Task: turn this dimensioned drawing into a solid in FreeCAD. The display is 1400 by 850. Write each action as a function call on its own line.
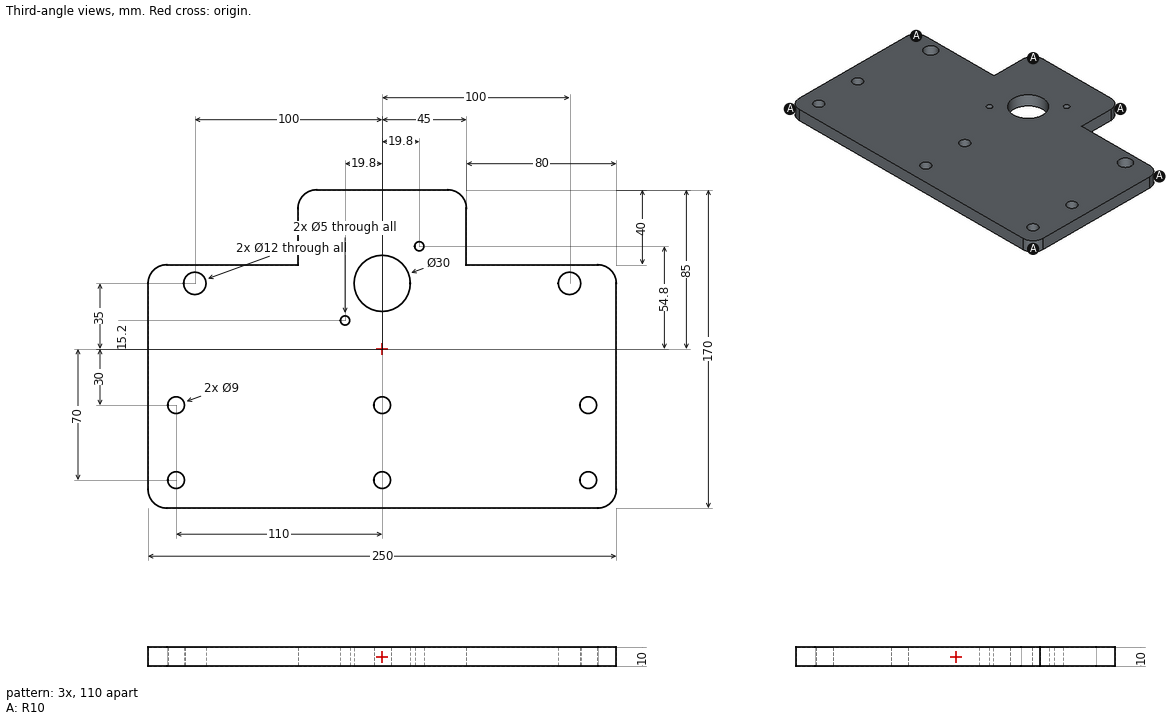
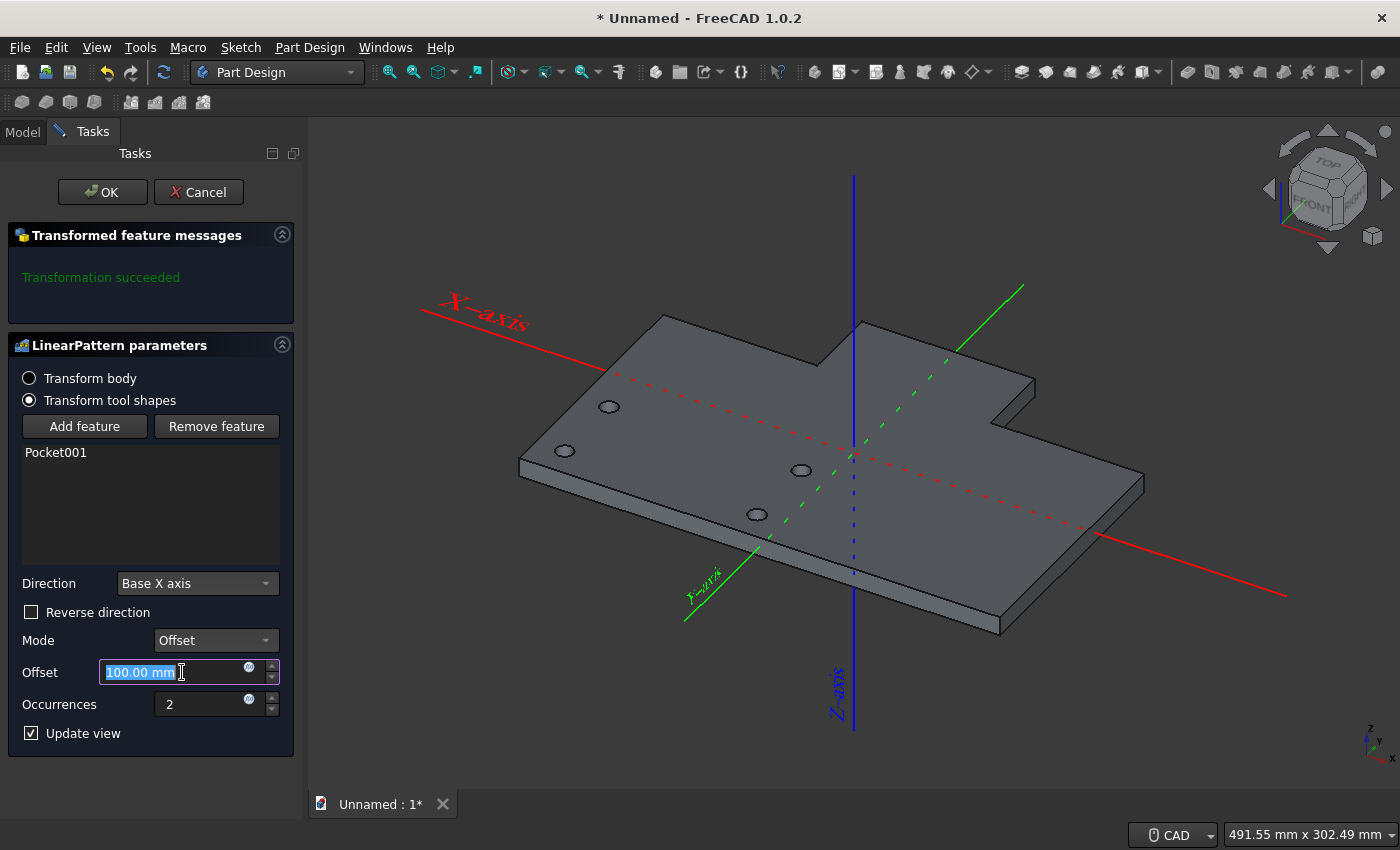
text(110)
key(Tab)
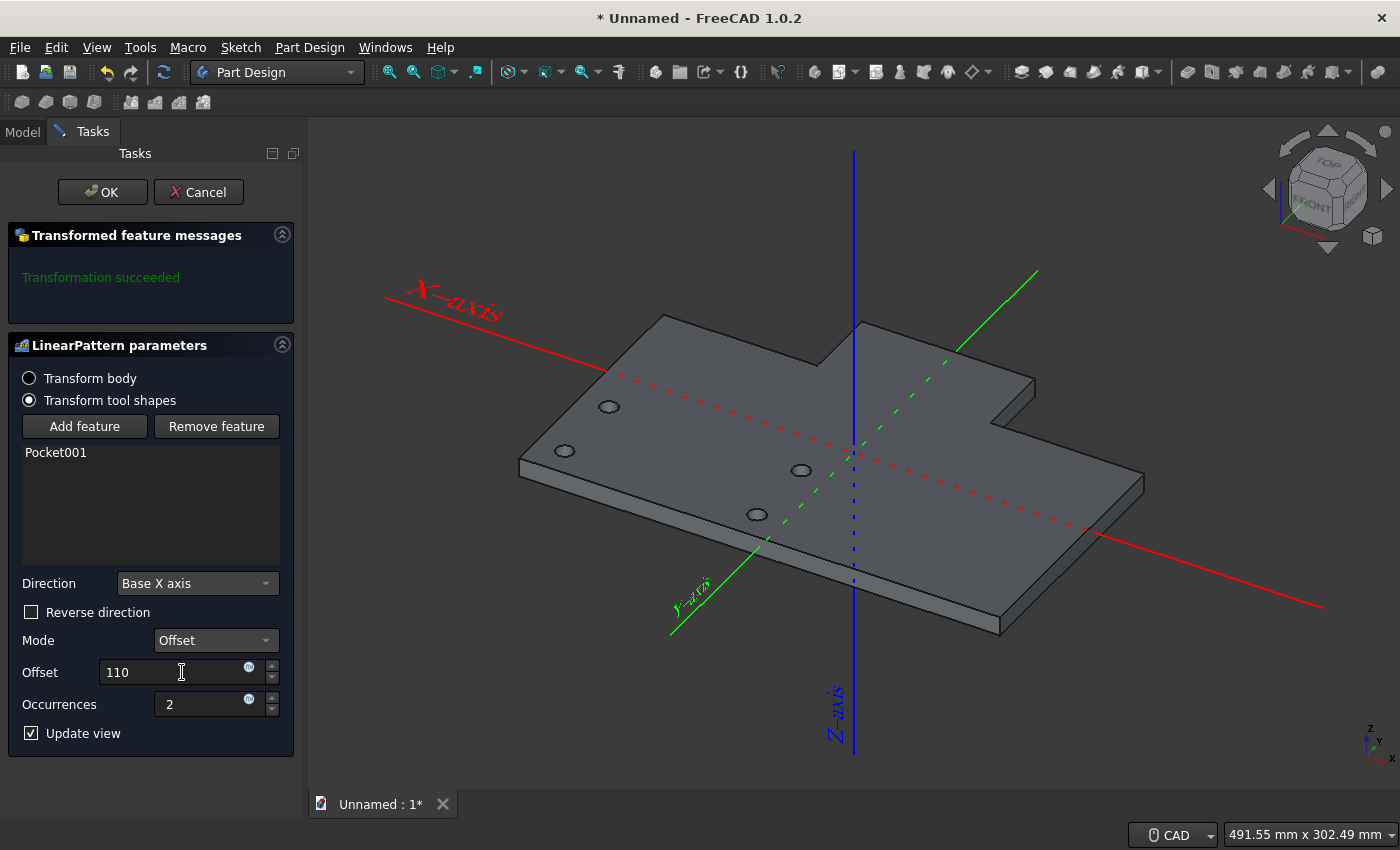
triple_click(209, 704)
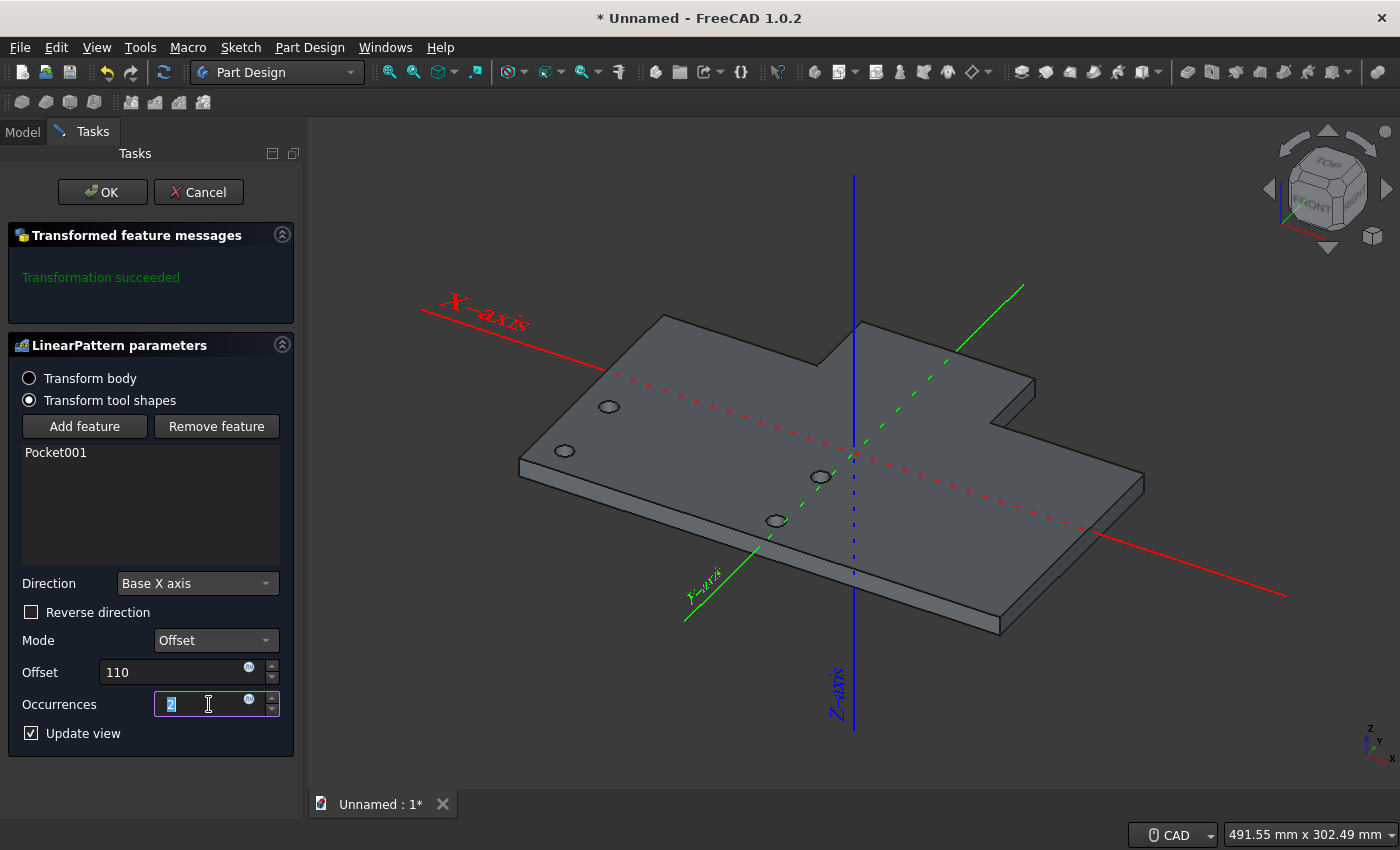
text(3)
key(Tab)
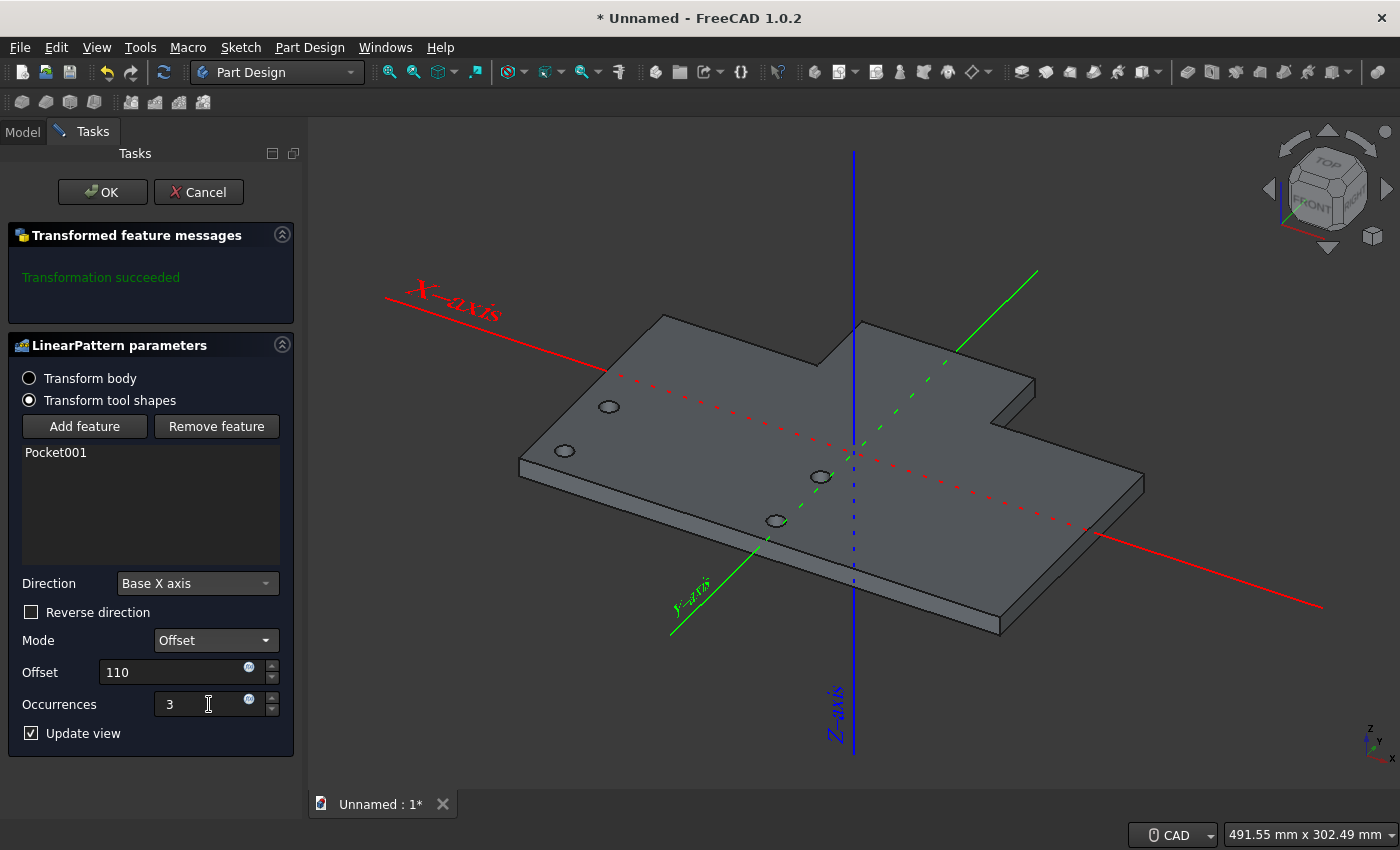
click(103, 192)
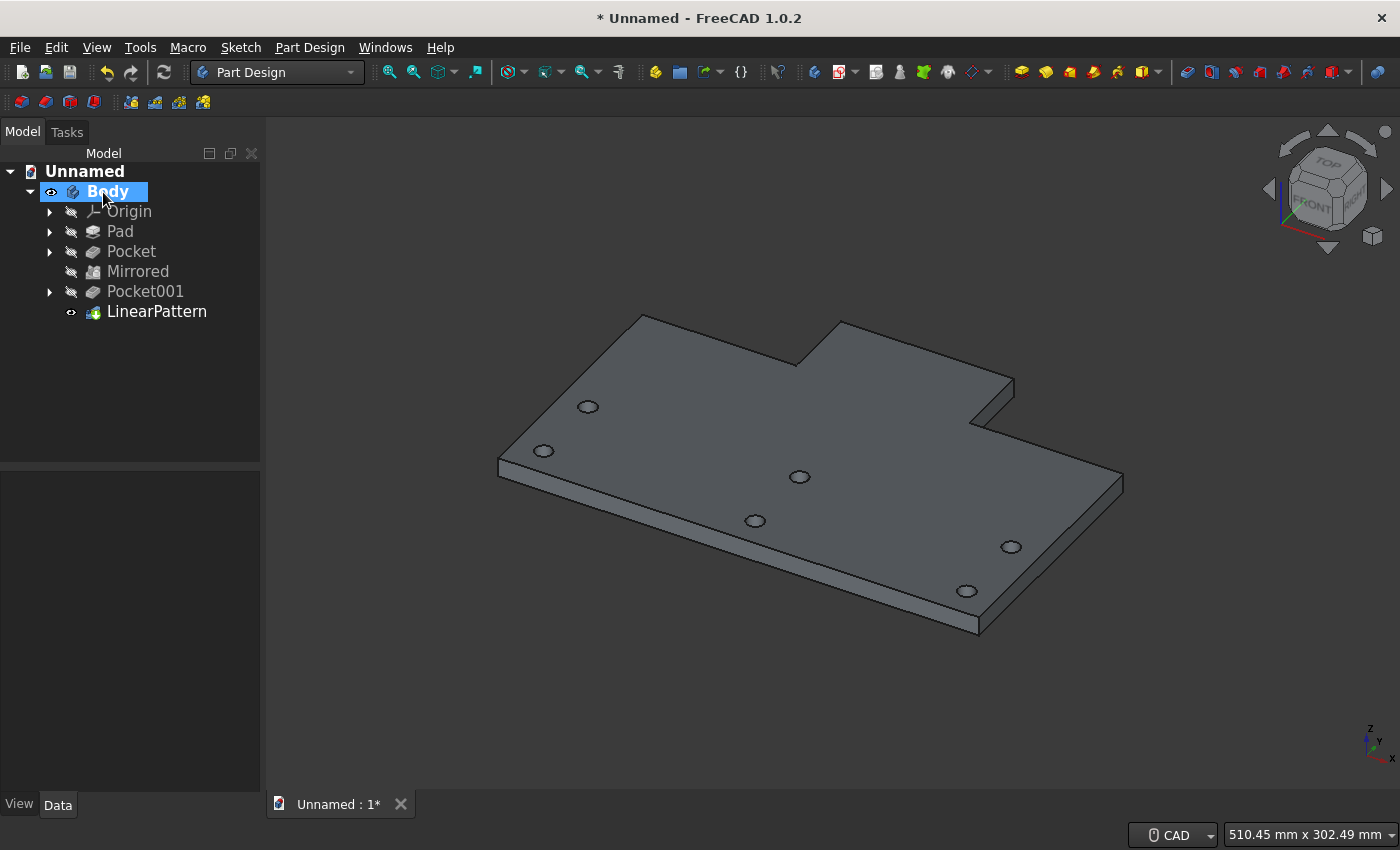
click(860, 416)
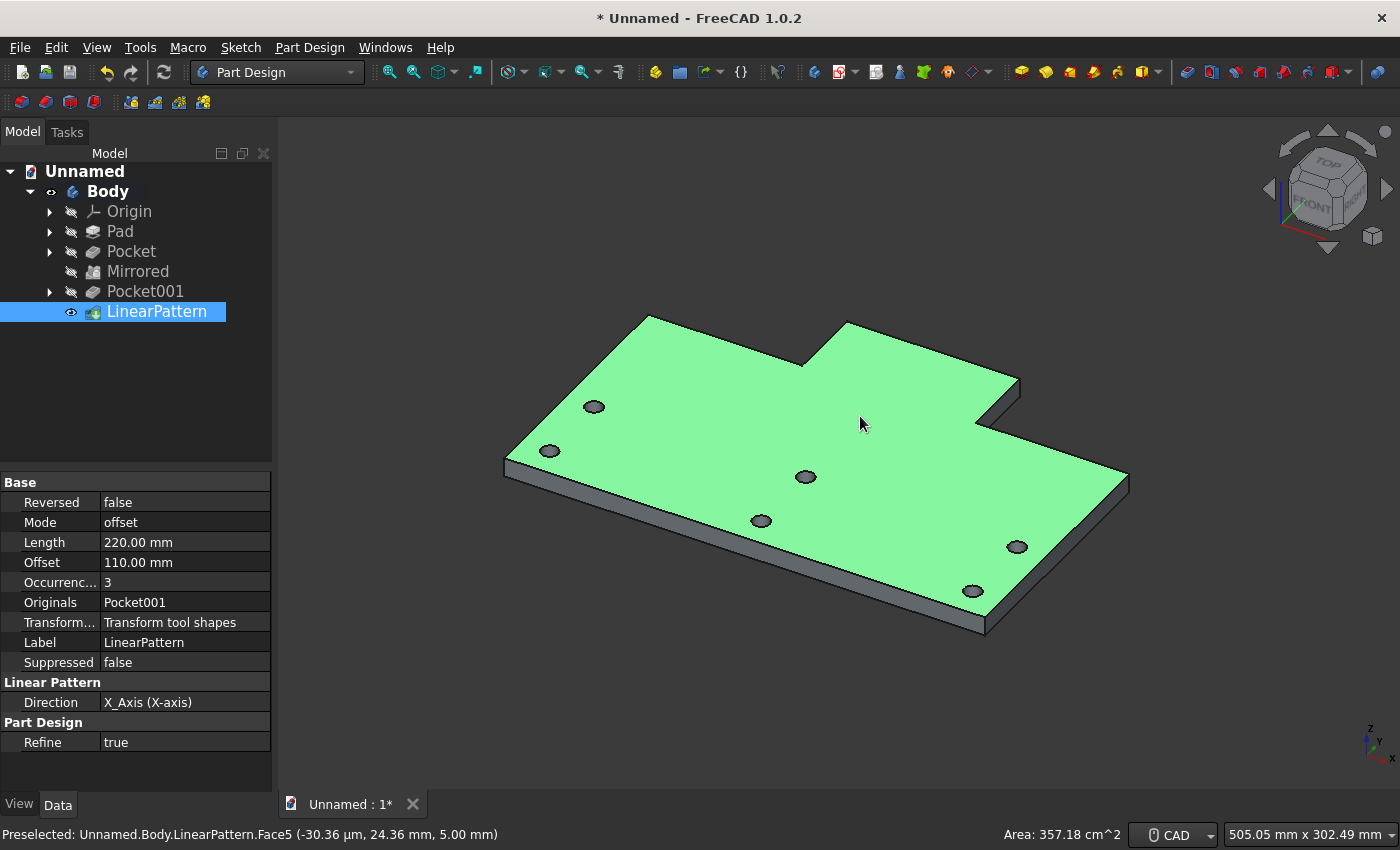
click(840, 72)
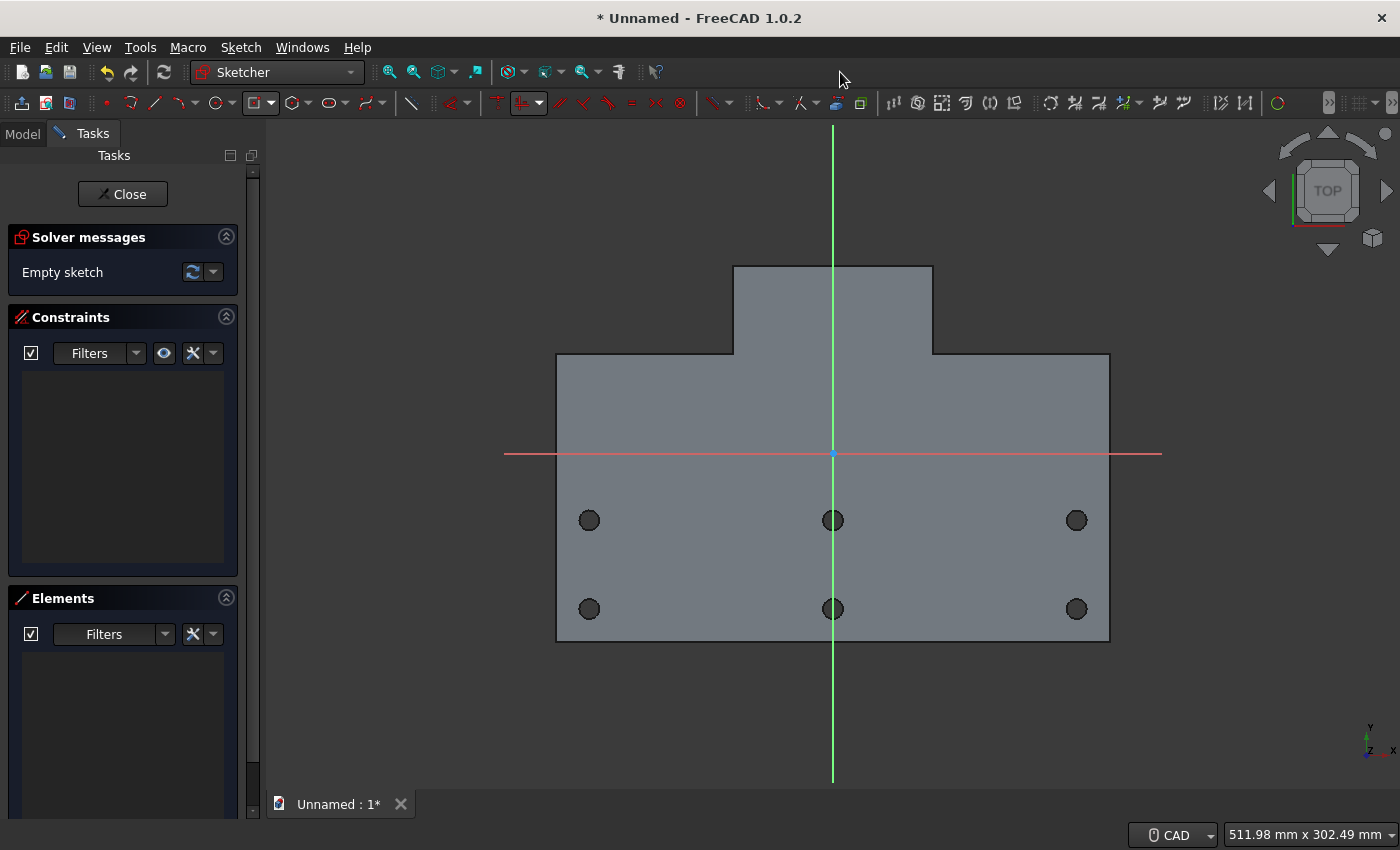
scroll(972, 316, up, 2)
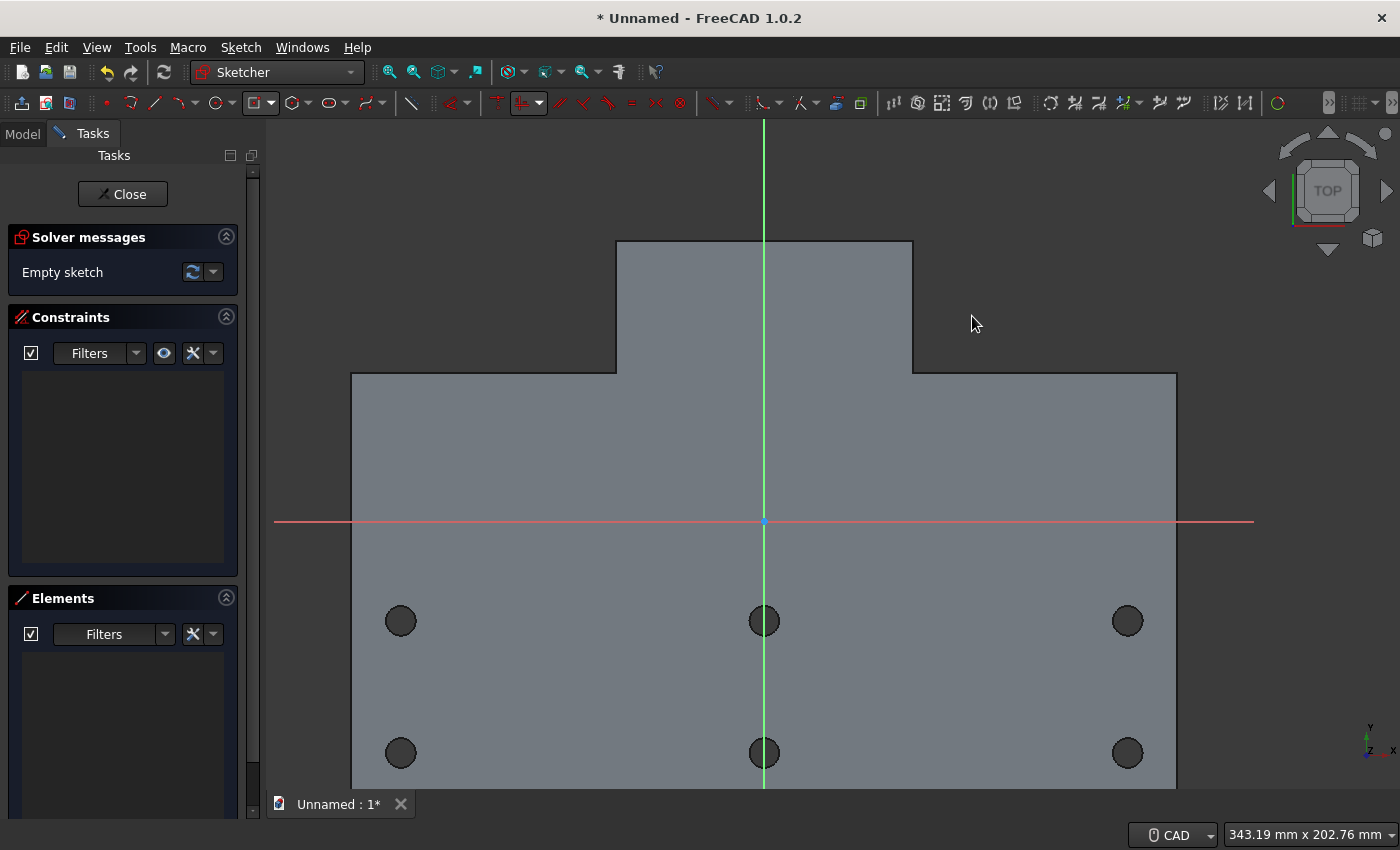
click(216, 104)